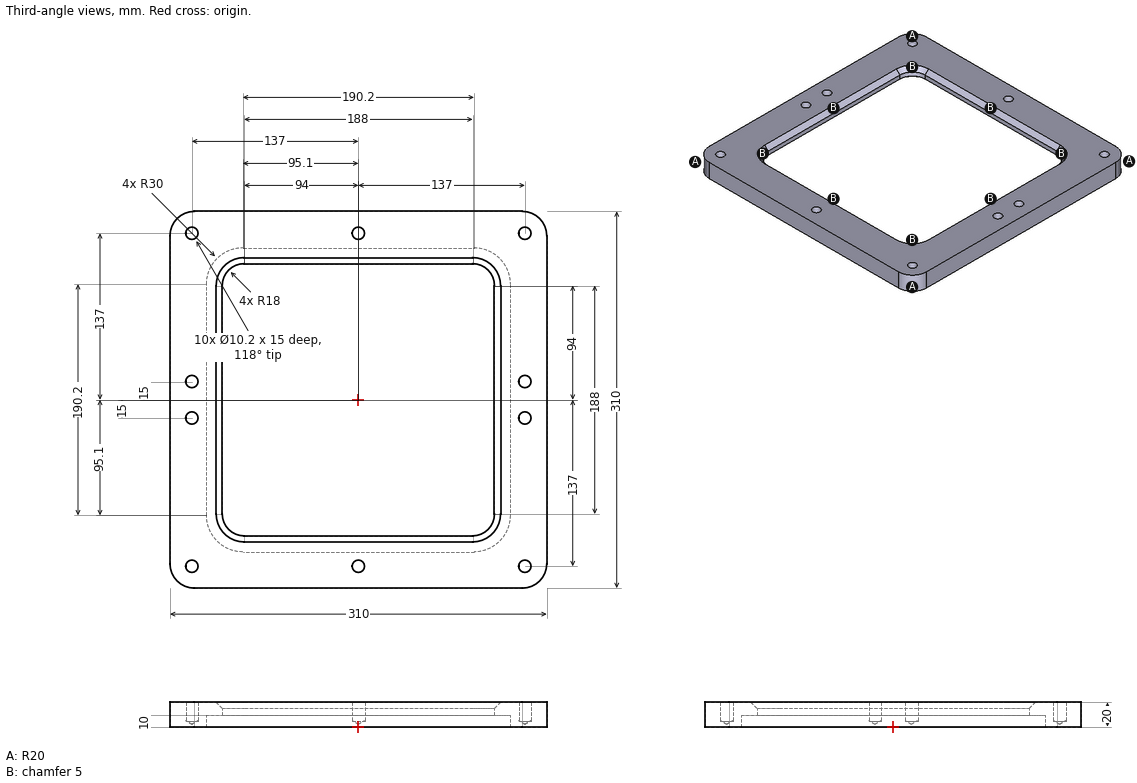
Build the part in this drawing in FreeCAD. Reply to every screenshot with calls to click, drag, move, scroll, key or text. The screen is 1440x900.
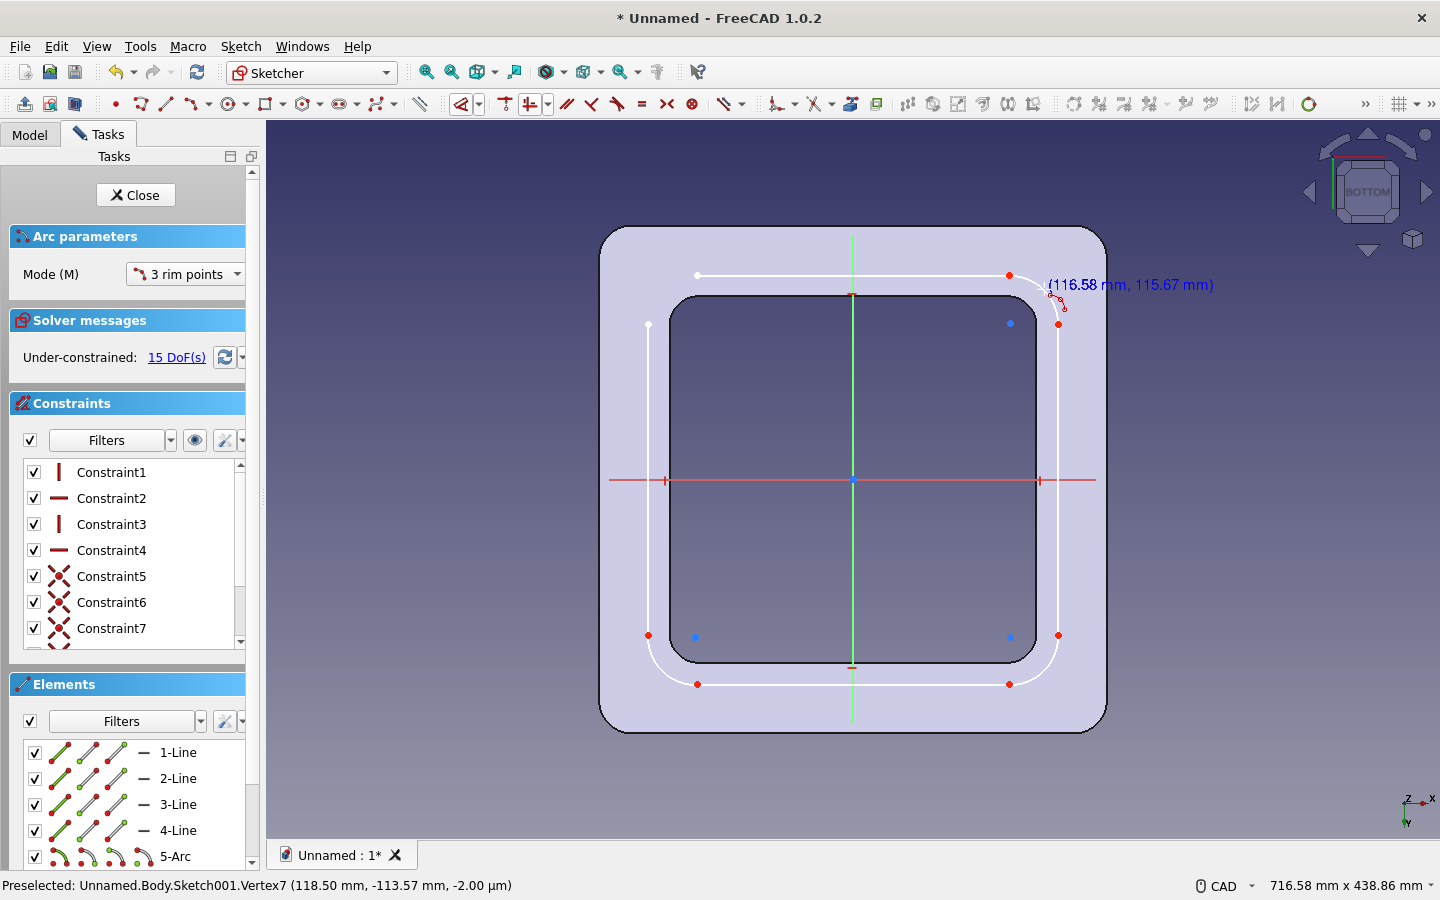
click(697, 276)
click(648, 325)
click(662, 289)
key(Escape)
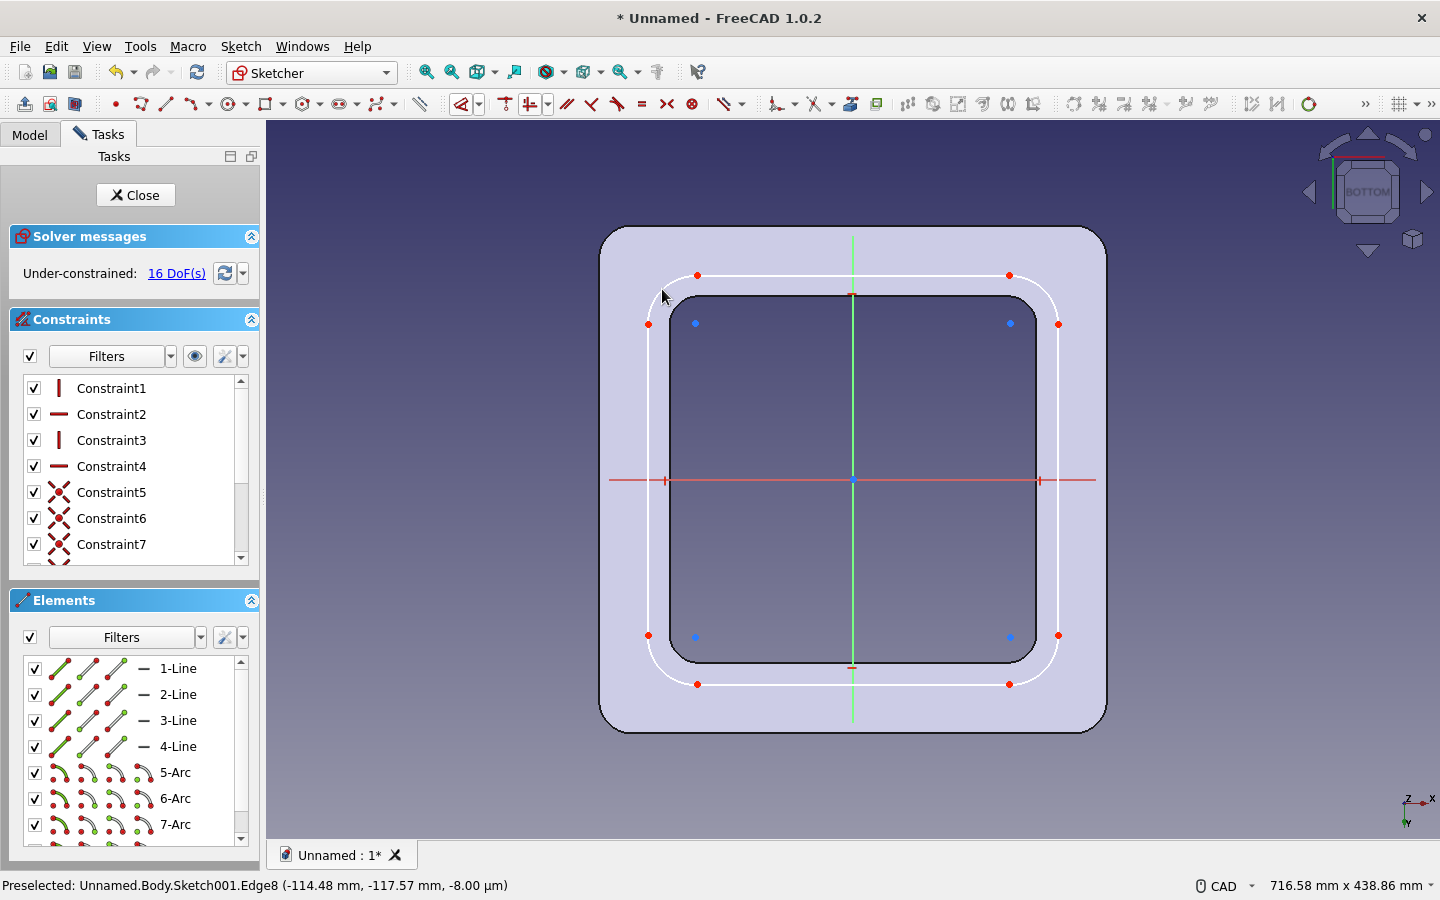
click(648, 418)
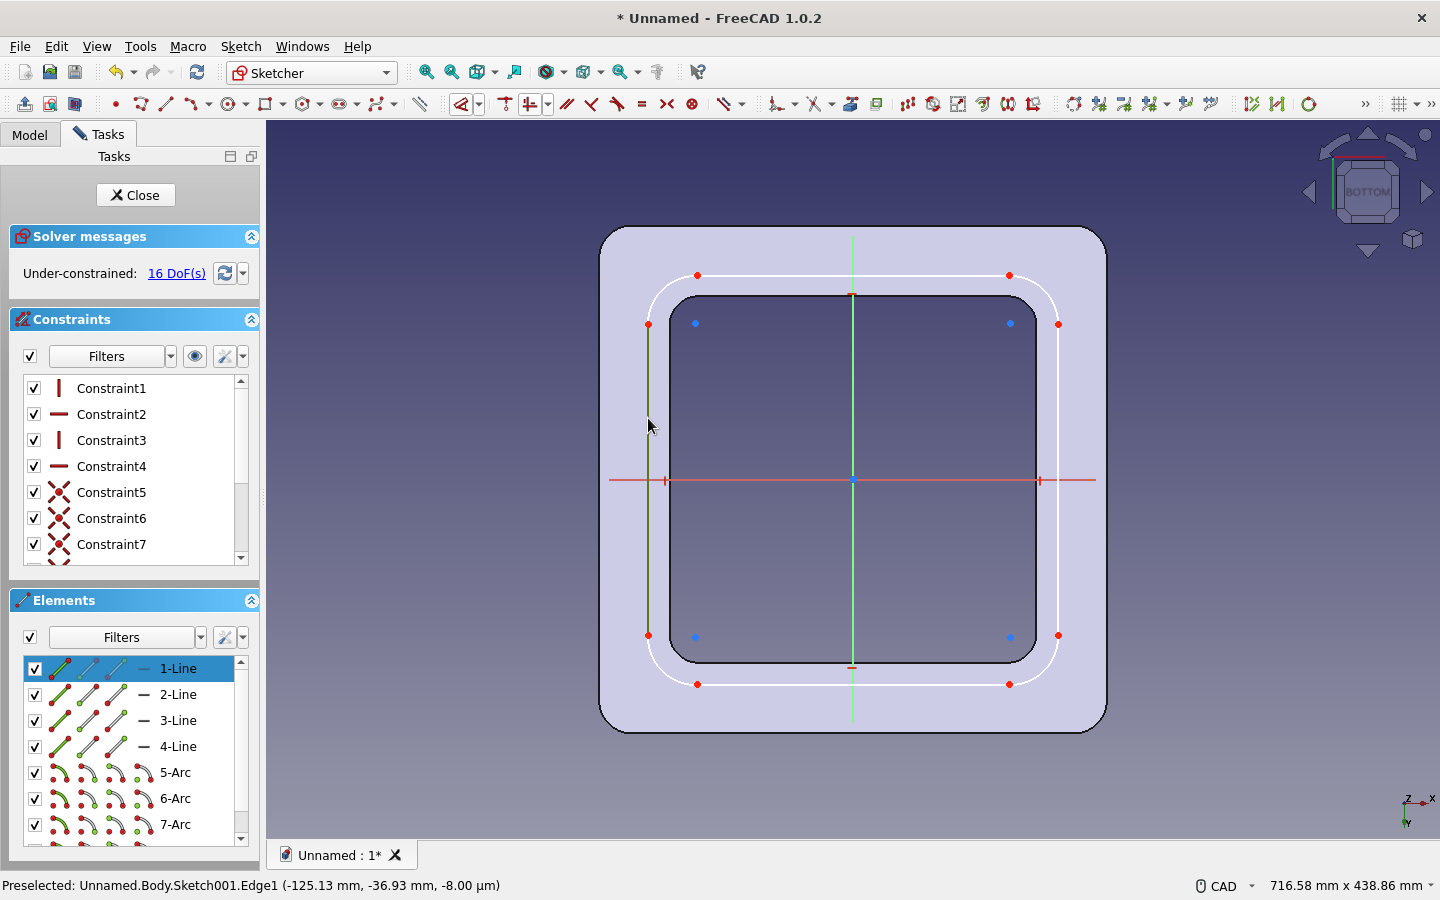
click(653, 658)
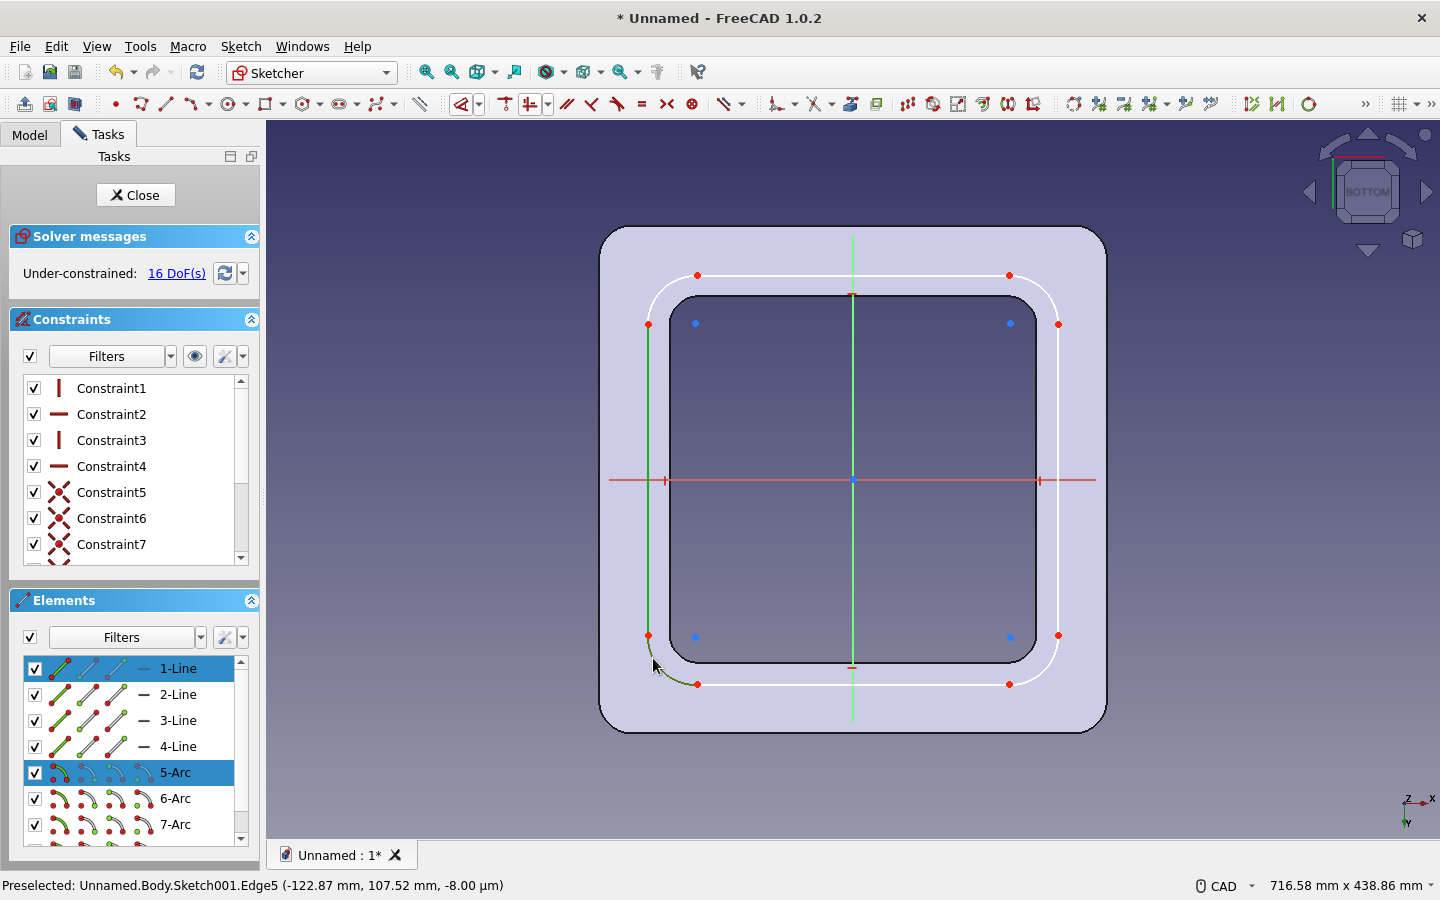
click(617, 104)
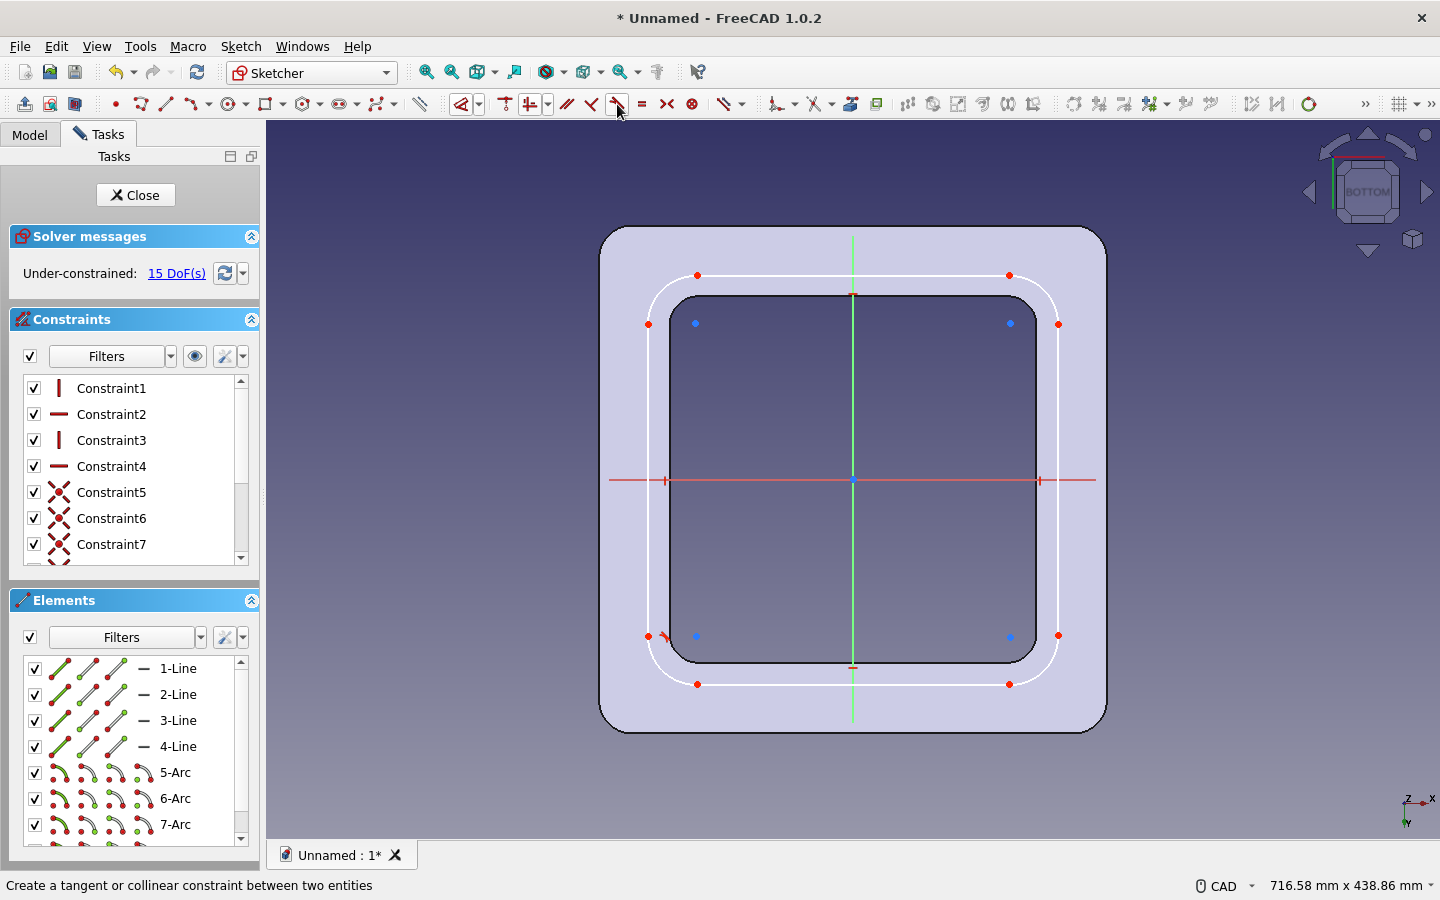
click(648, 418)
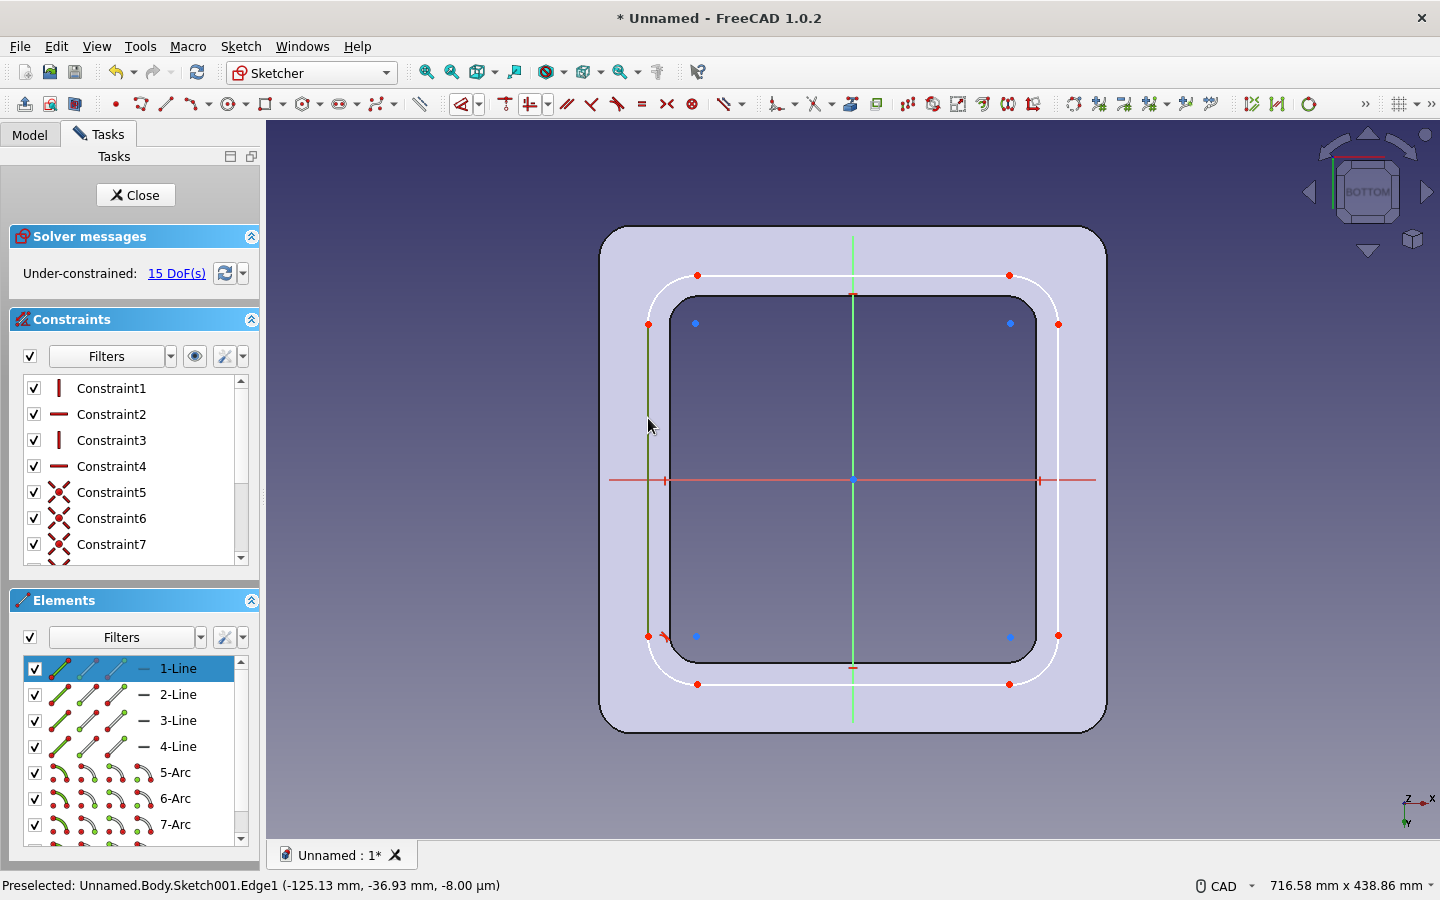
click(675, 281)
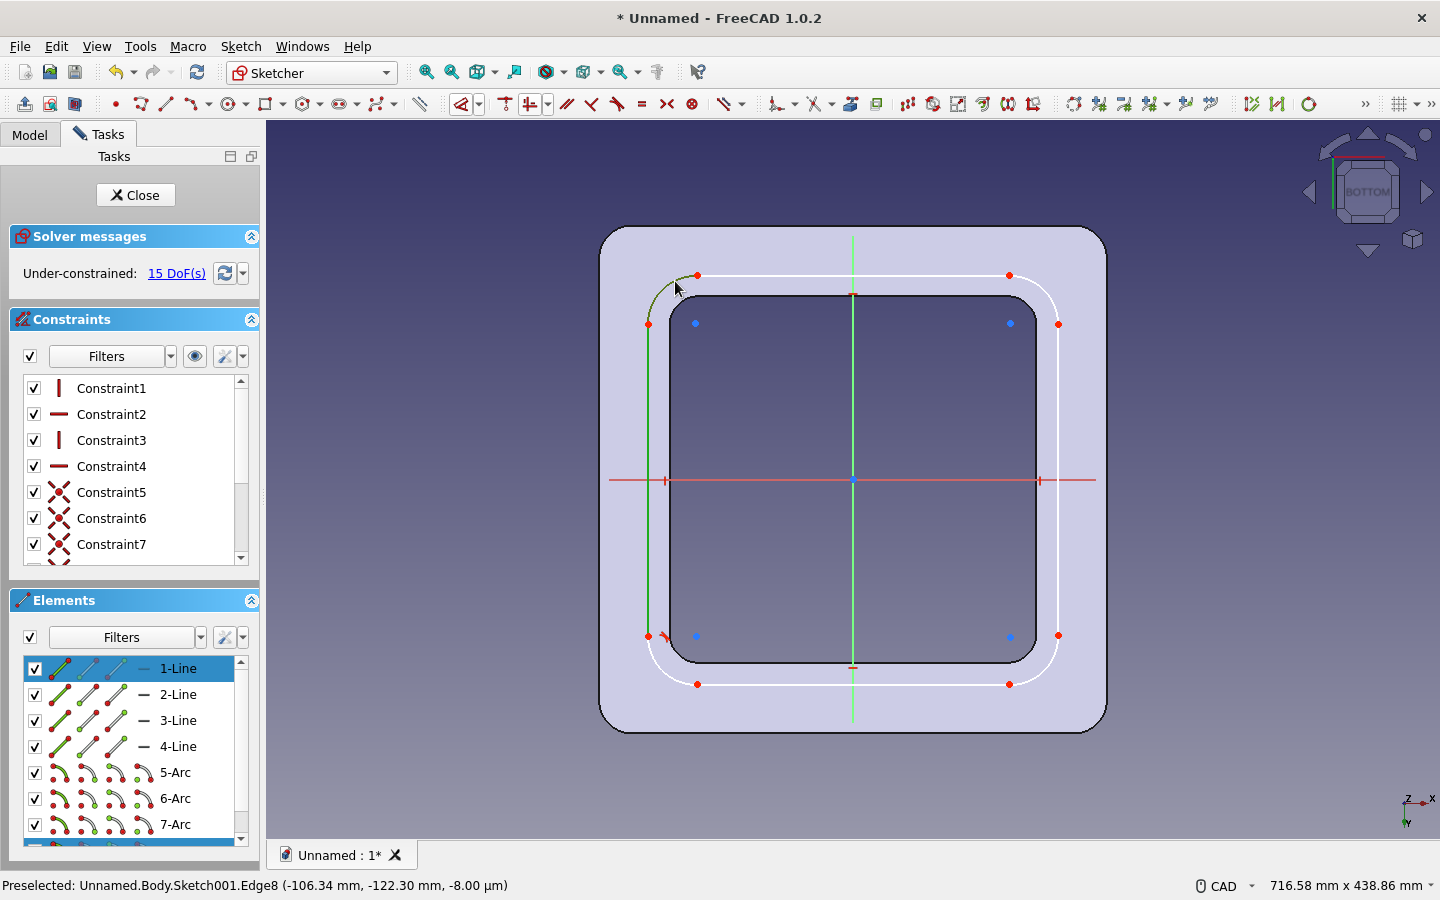
click(617, 104)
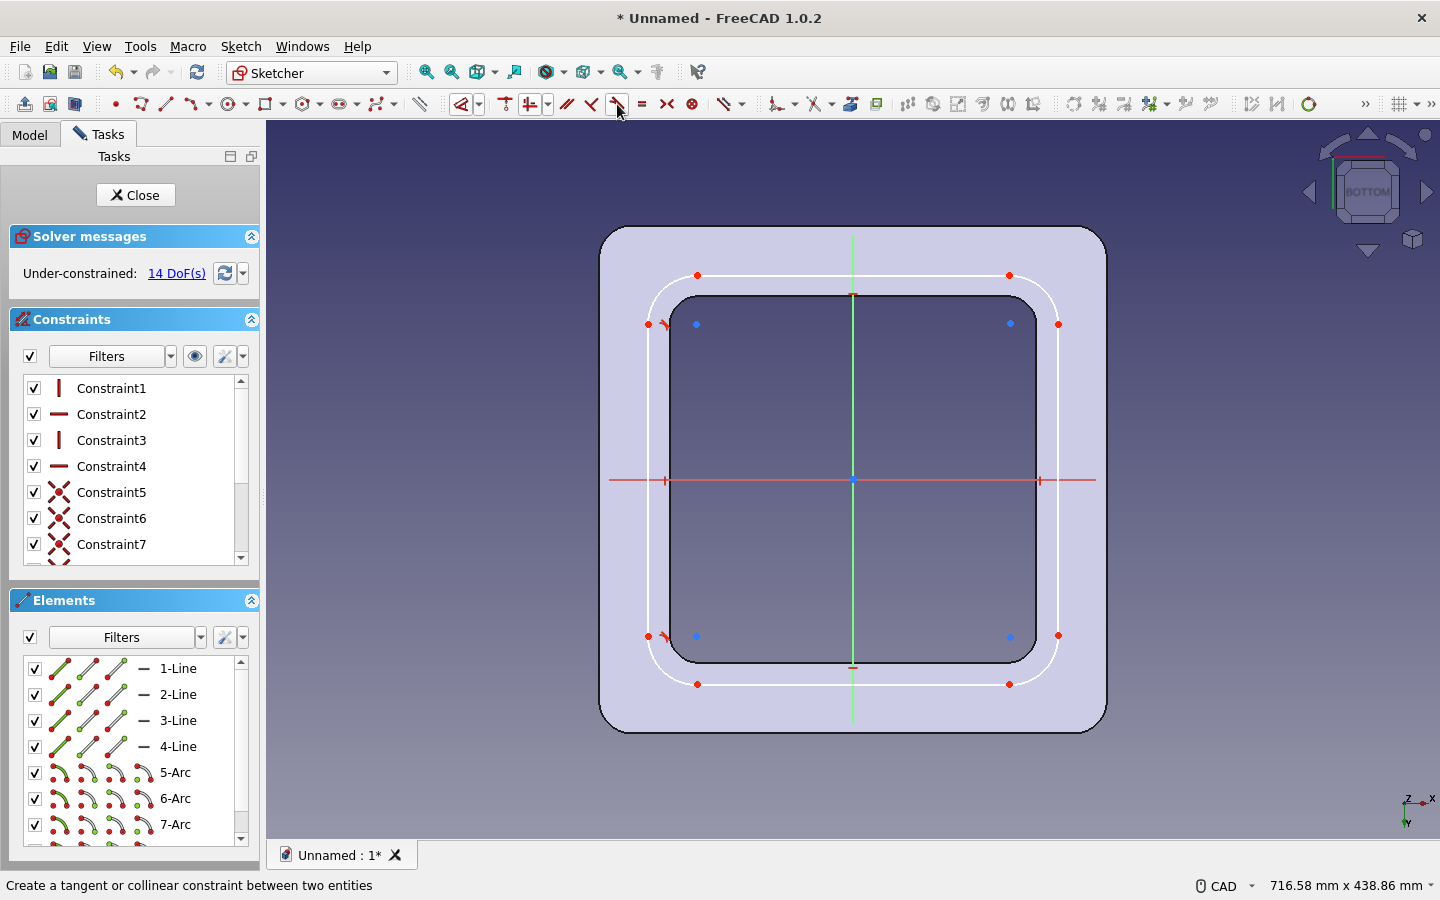
click(791, 685)